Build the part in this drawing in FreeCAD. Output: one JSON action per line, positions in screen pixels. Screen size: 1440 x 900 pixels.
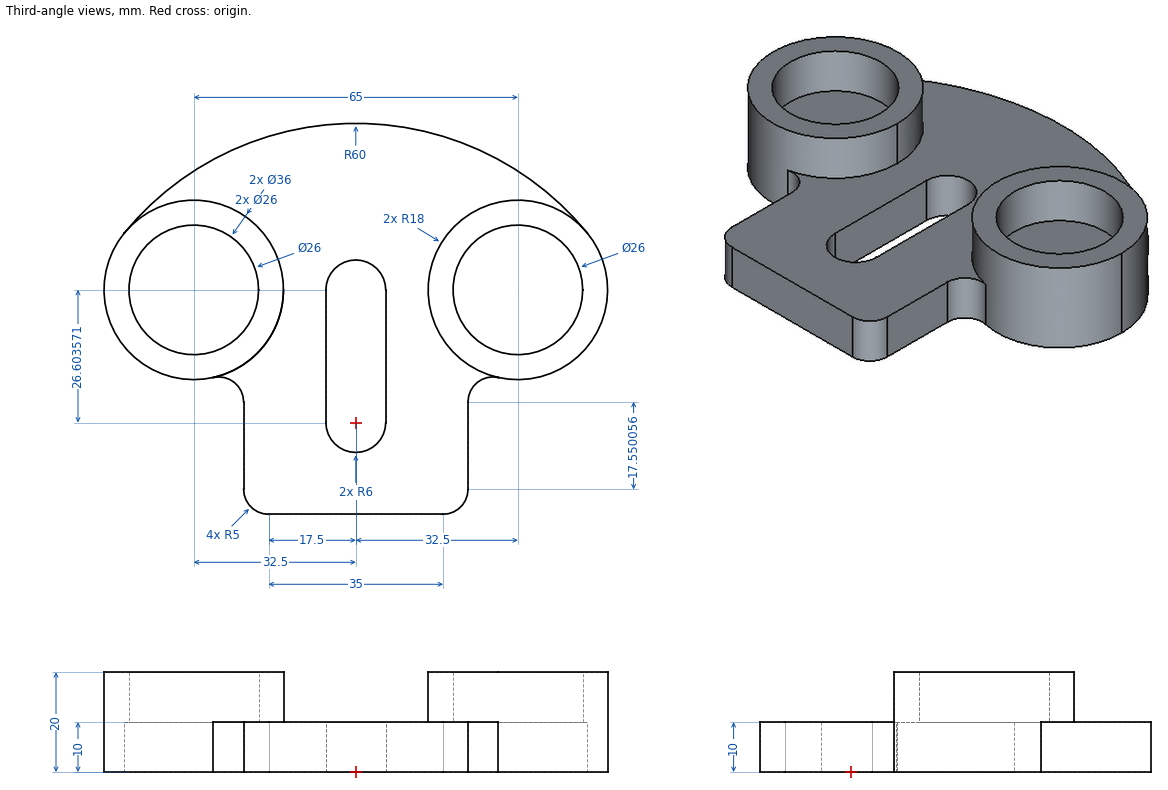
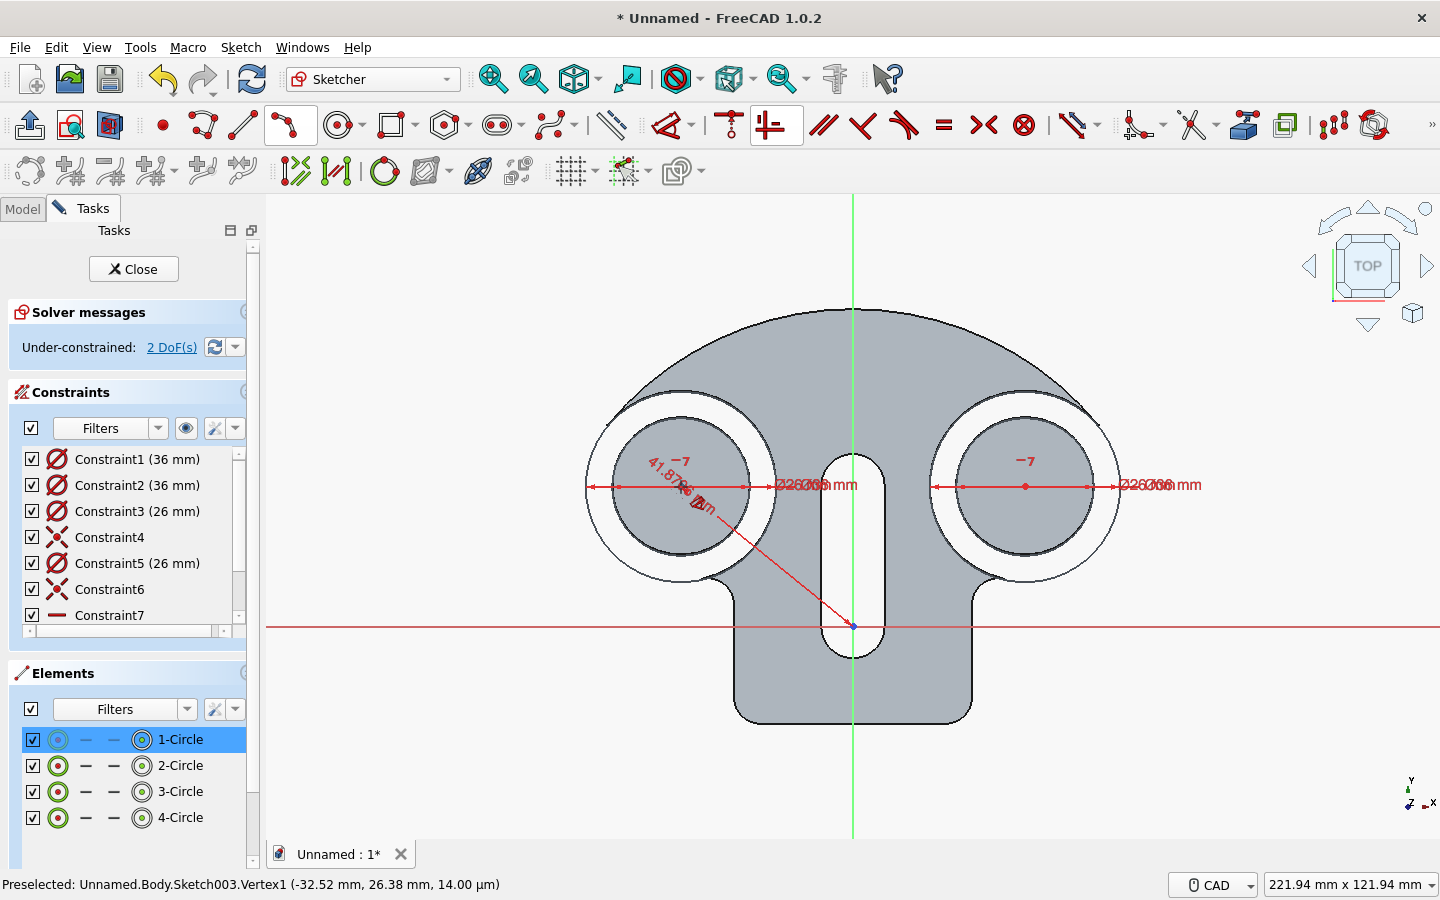
{"action": "left_click", "coordinate": [1025, 487]}
{"action": "left_click", "coordinate": [774, 429]}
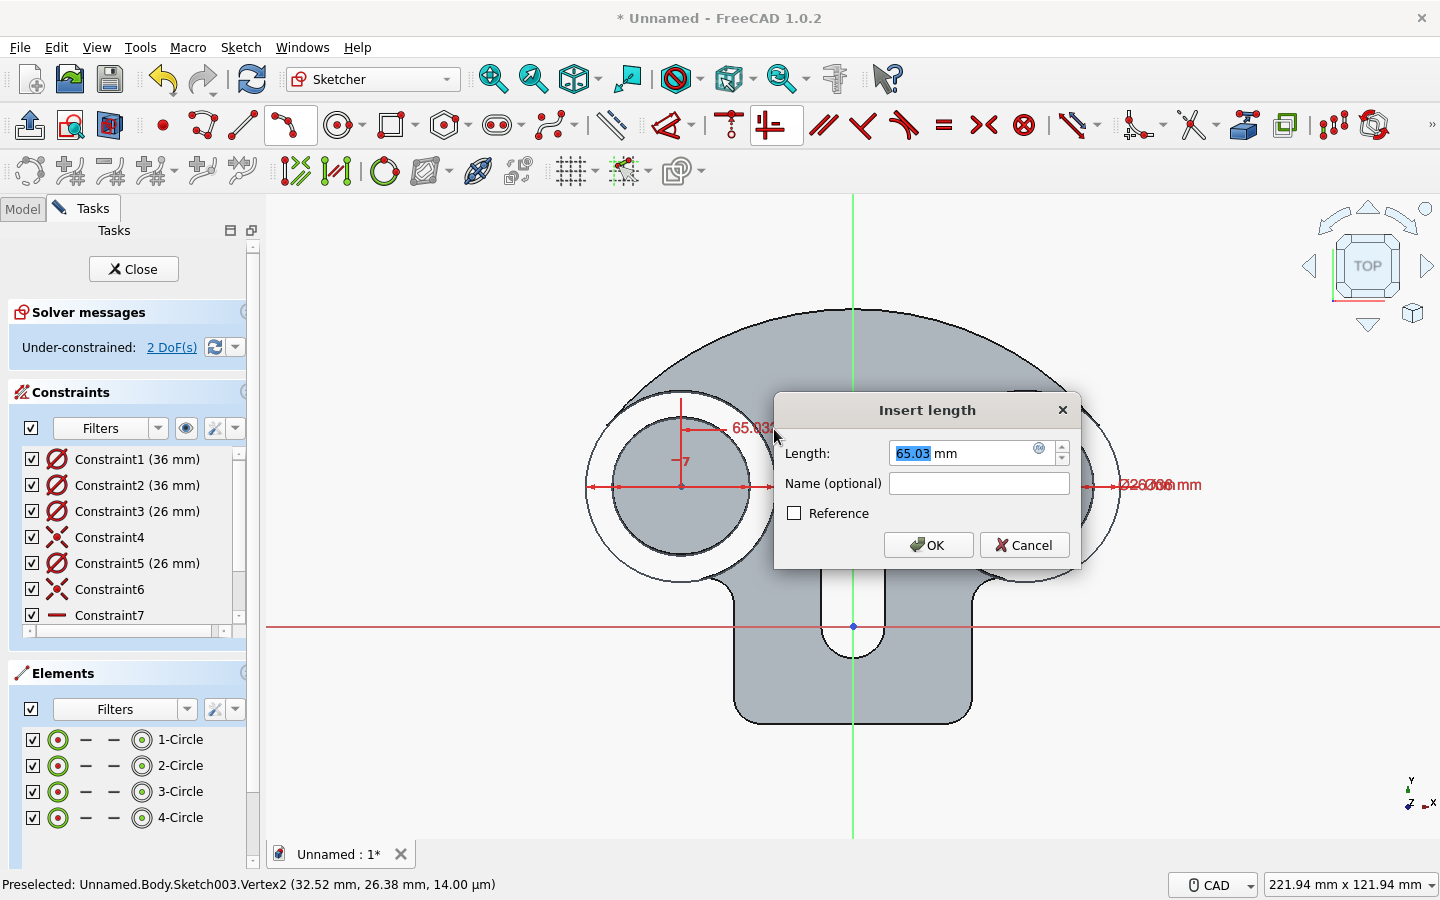
{"action": "type", "text": "65"}
{"action": "key", "text": "Return"}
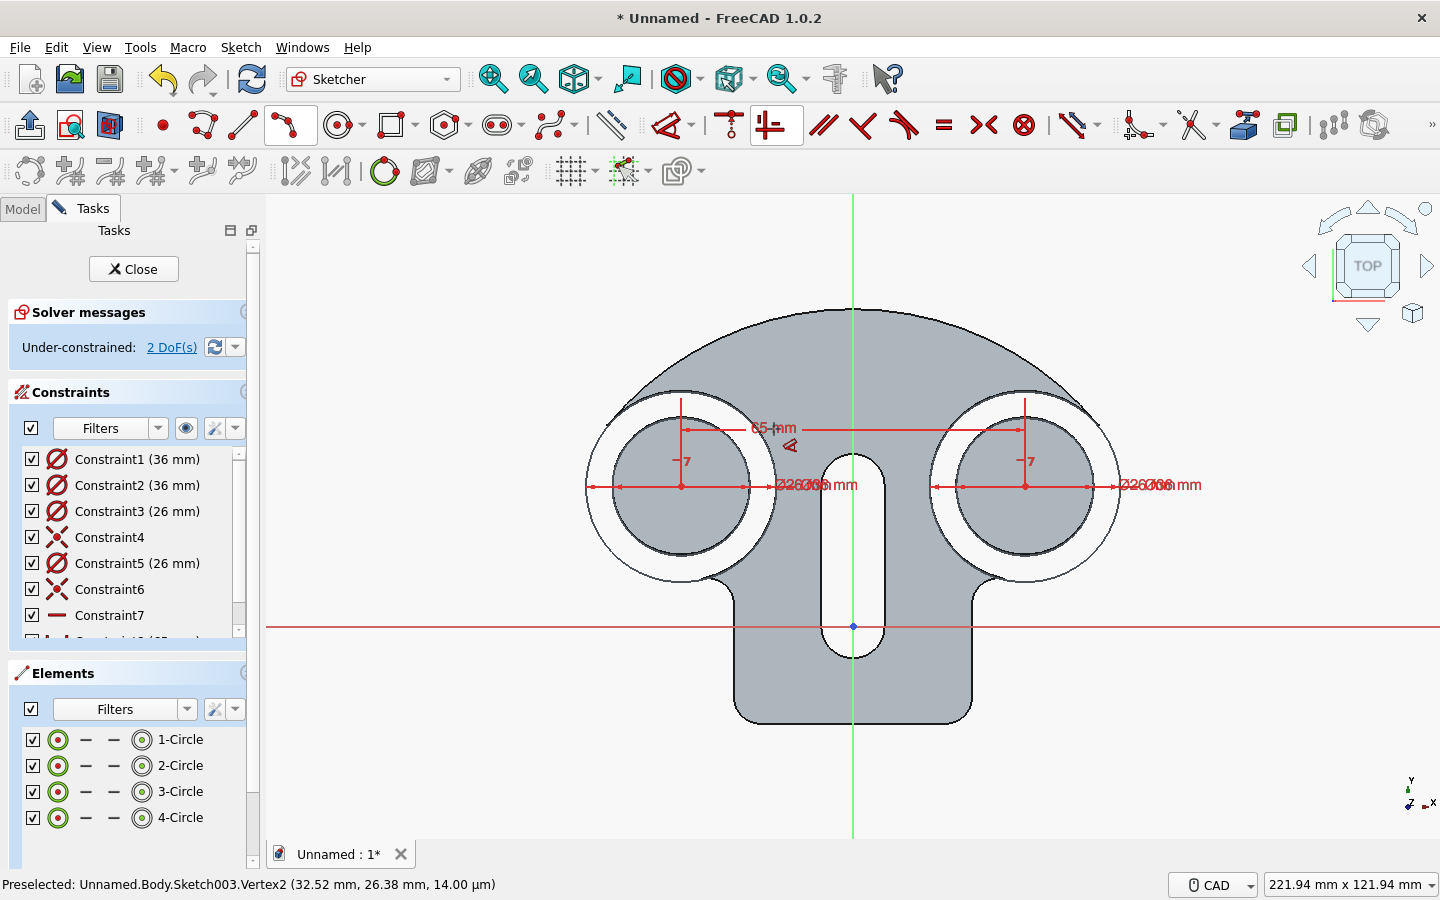
{"action": "left_click", "coordinate": [681, 487]}
{"action": "left_click", "coordinate": [767, 661]}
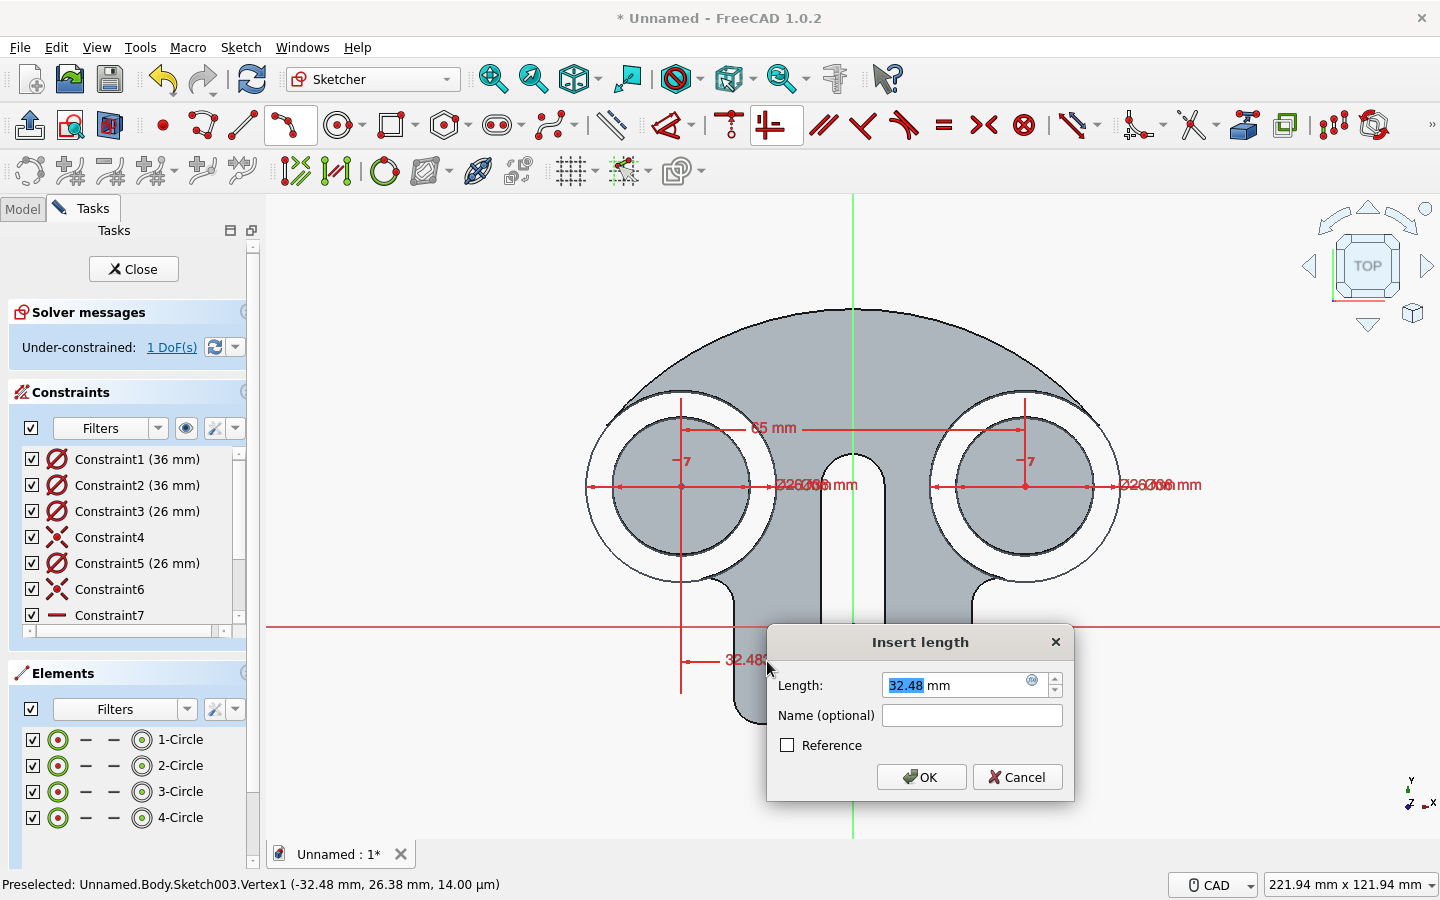
{"action": "type", "text": "32.5"}
{"action": "key", "text": "Return"}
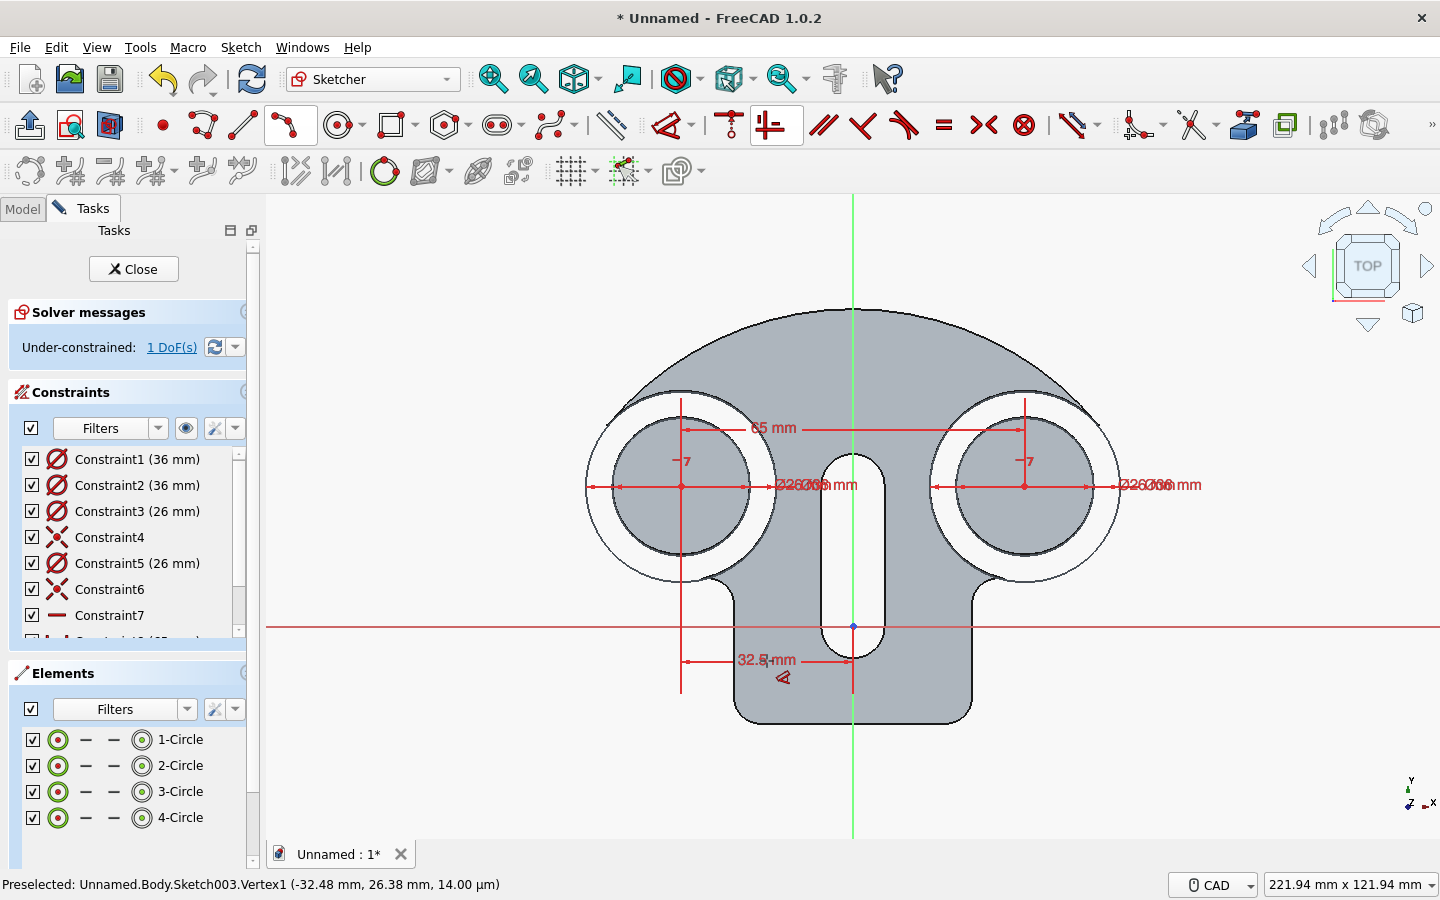
{"action": "left_click", "coordinate": [681, 487]}
{"action": "left_click", "coordinate": [647, 525]}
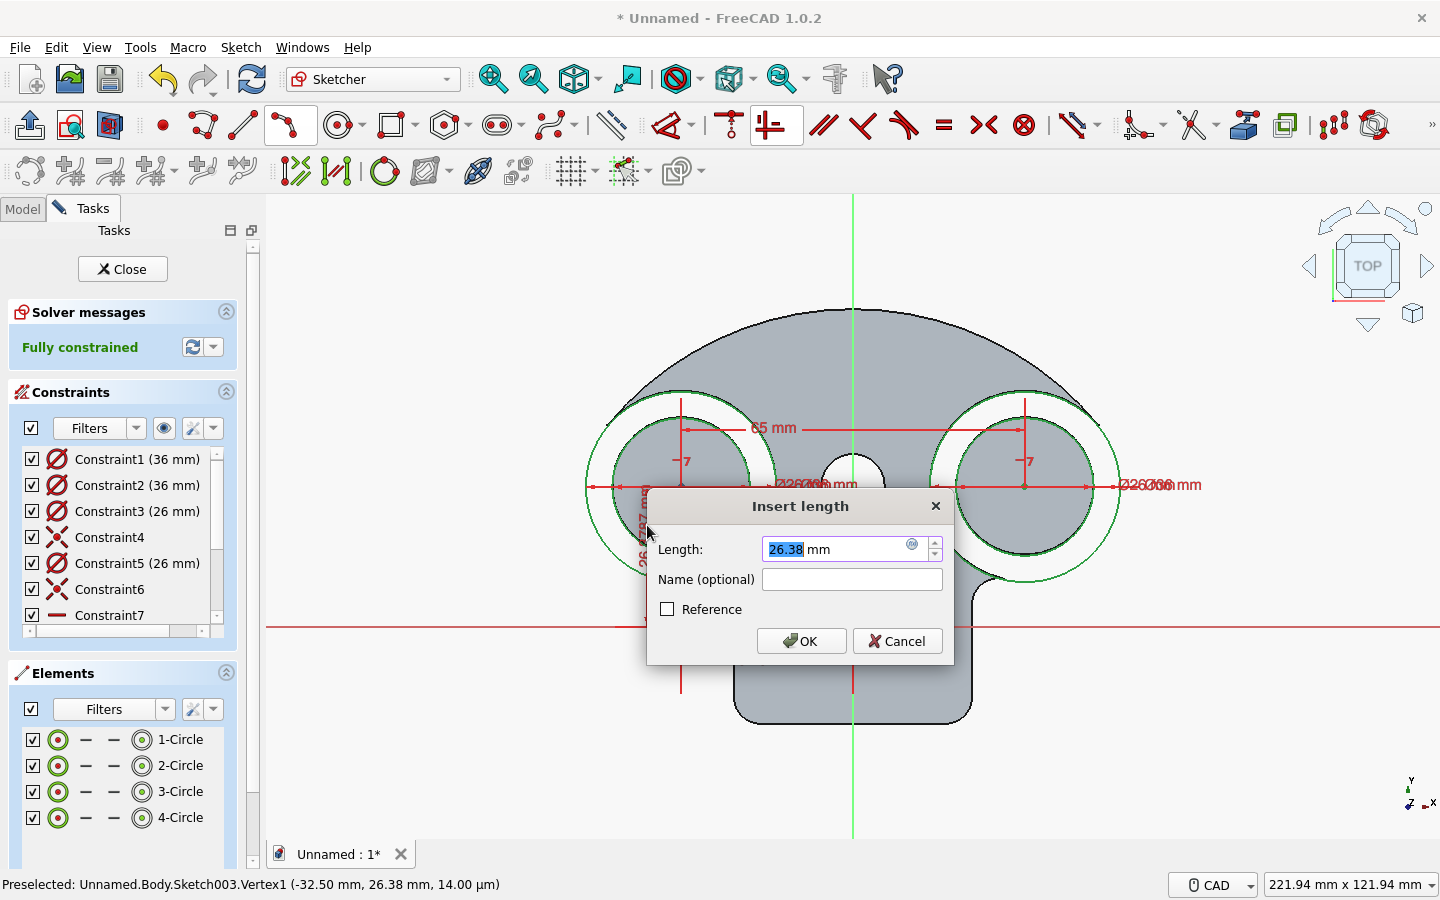
{"action": "type", "text": "26.603571"}
{"action": "key", "text": "Return"}
{"action": "key", "text": "Escape"}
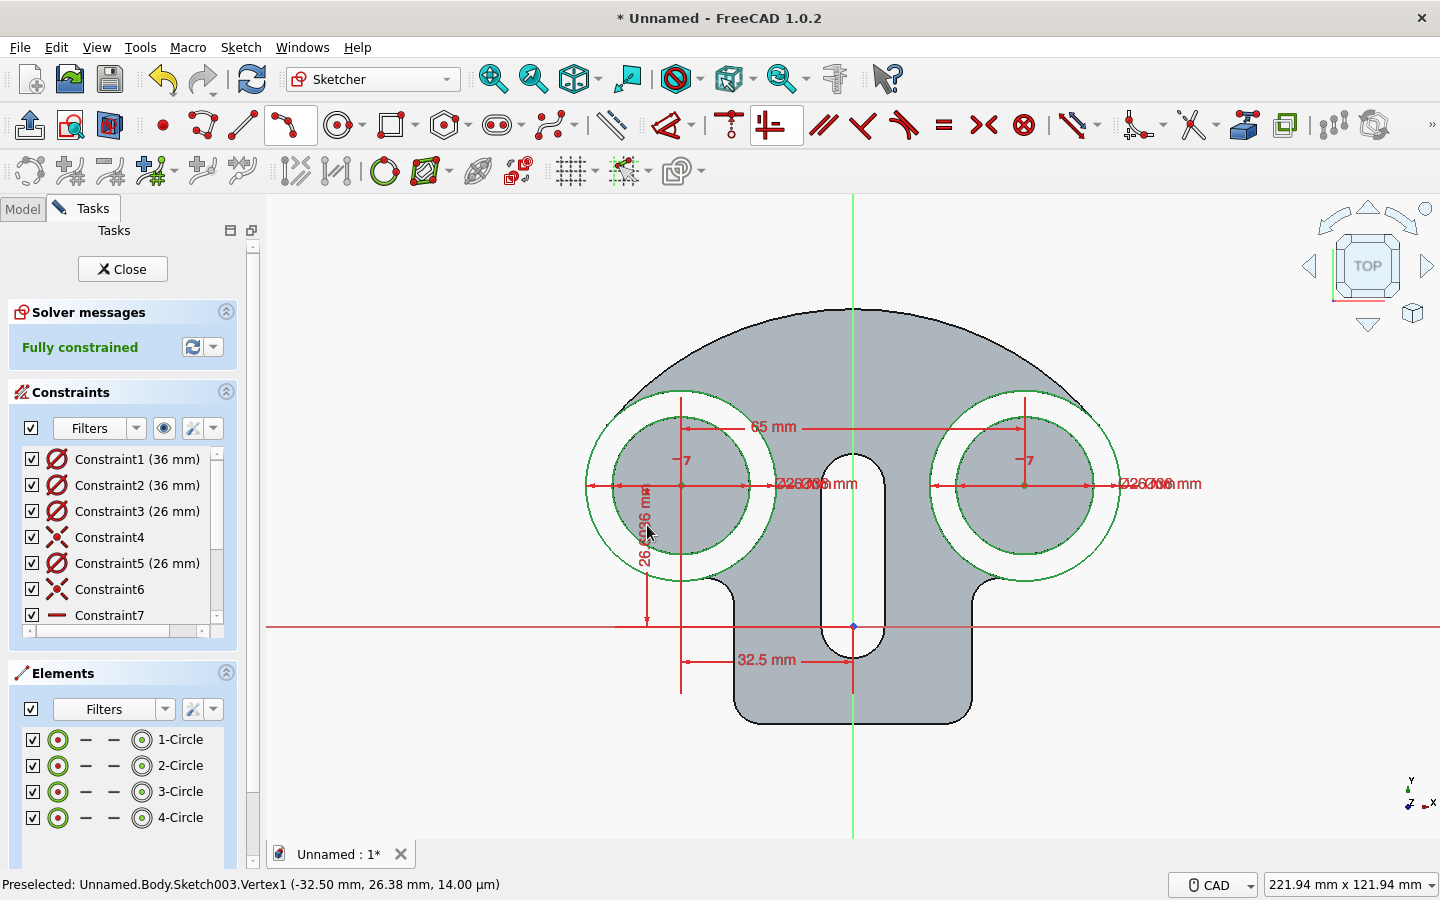
{"action": "left_click", "coordinate": [123, 269]}